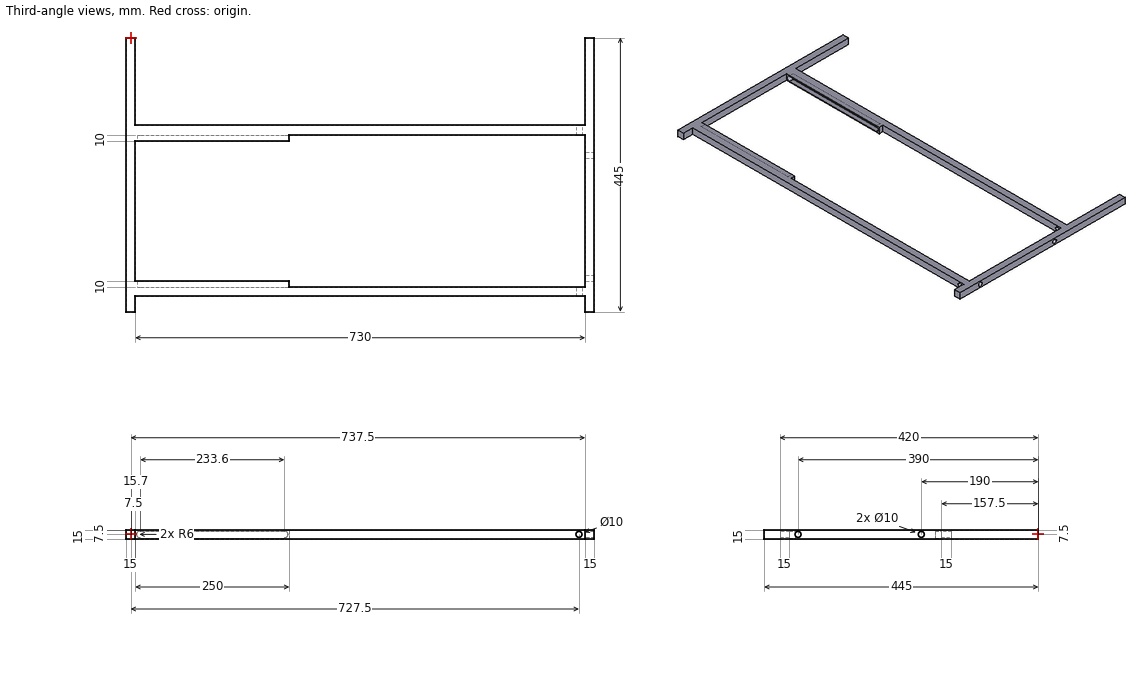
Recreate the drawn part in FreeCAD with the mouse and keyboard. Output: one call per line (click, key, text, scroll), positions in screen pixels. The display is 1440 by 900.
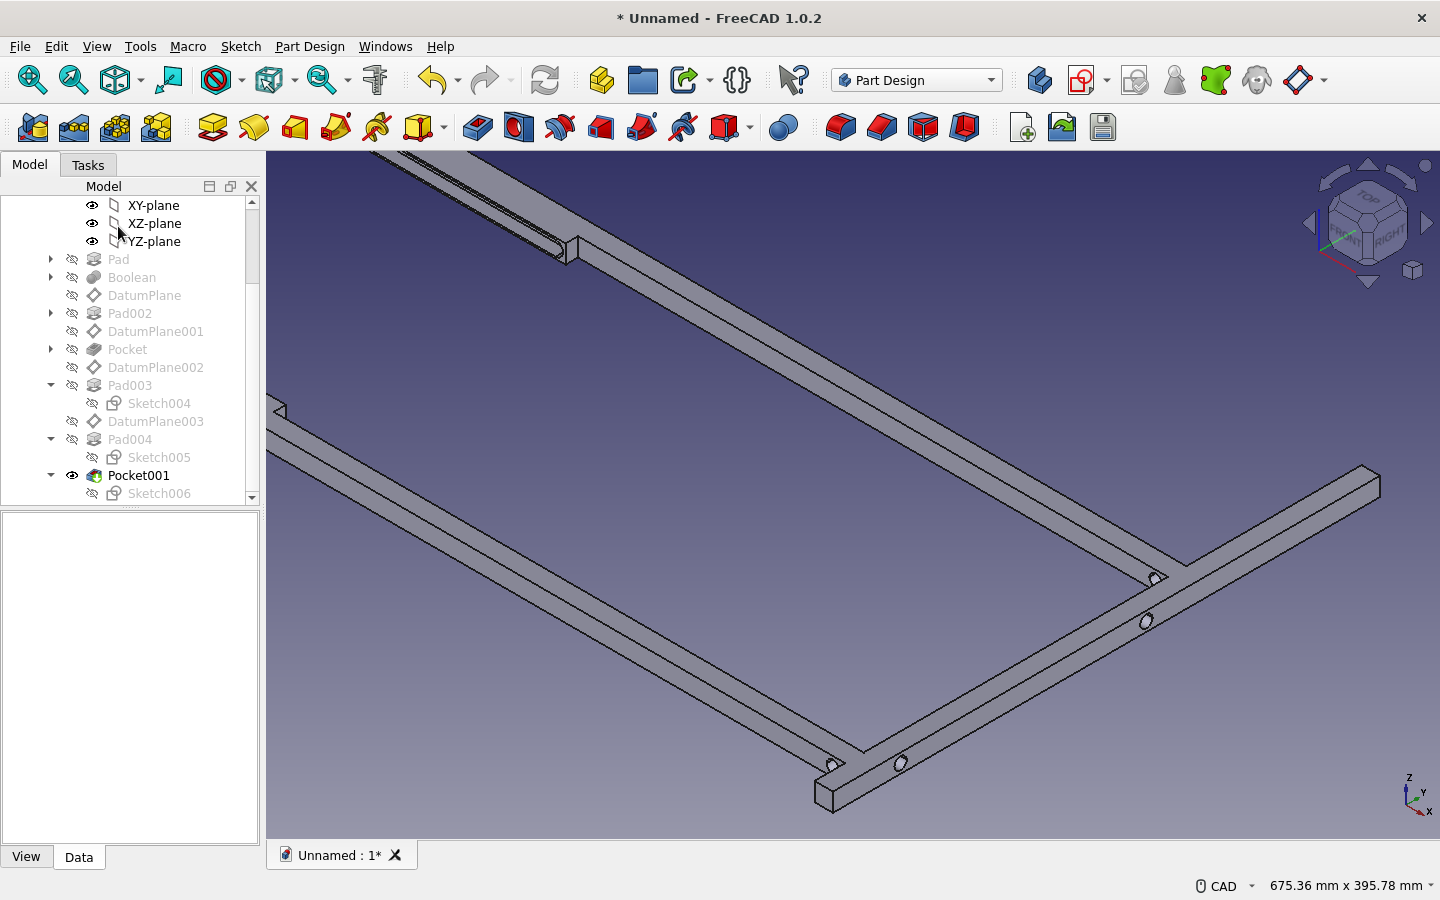
click(33, 80)